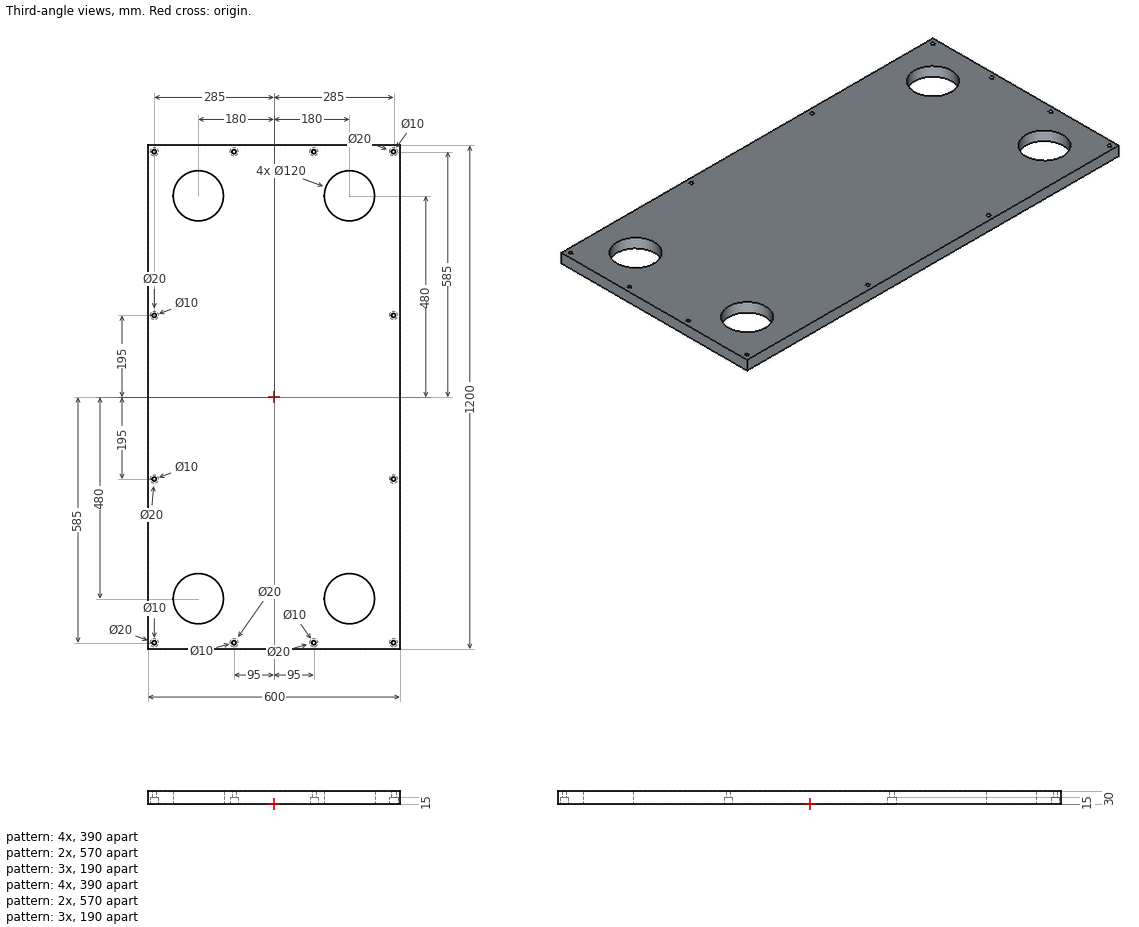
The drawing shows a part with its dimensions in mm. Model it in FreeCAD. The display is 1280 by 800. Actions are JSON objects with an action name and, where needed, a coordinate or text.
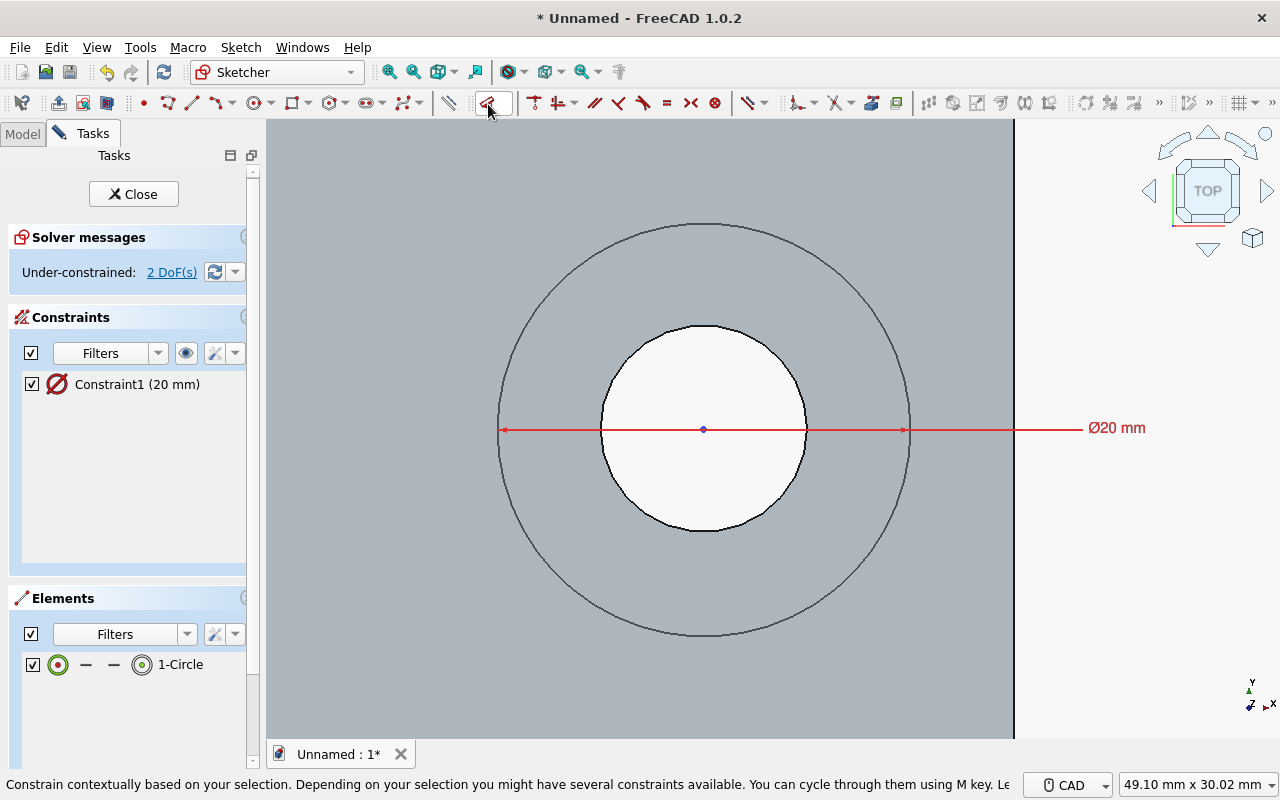
{"action": "left_click", "coordinate": [704, 430]}
{"action": "left_click", "coordinate": [405, 396]}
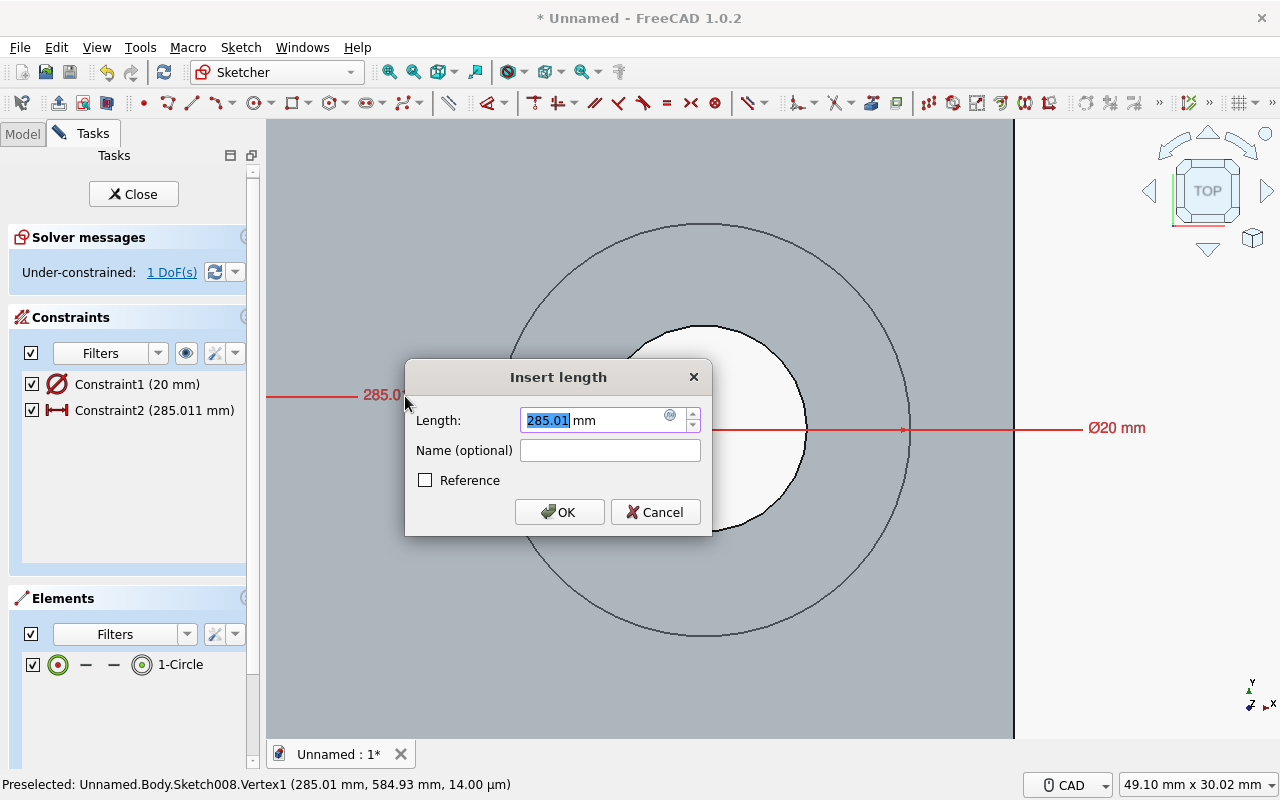
{"action": "type", "text": "285"}
{"action": "key", "text": "Return"}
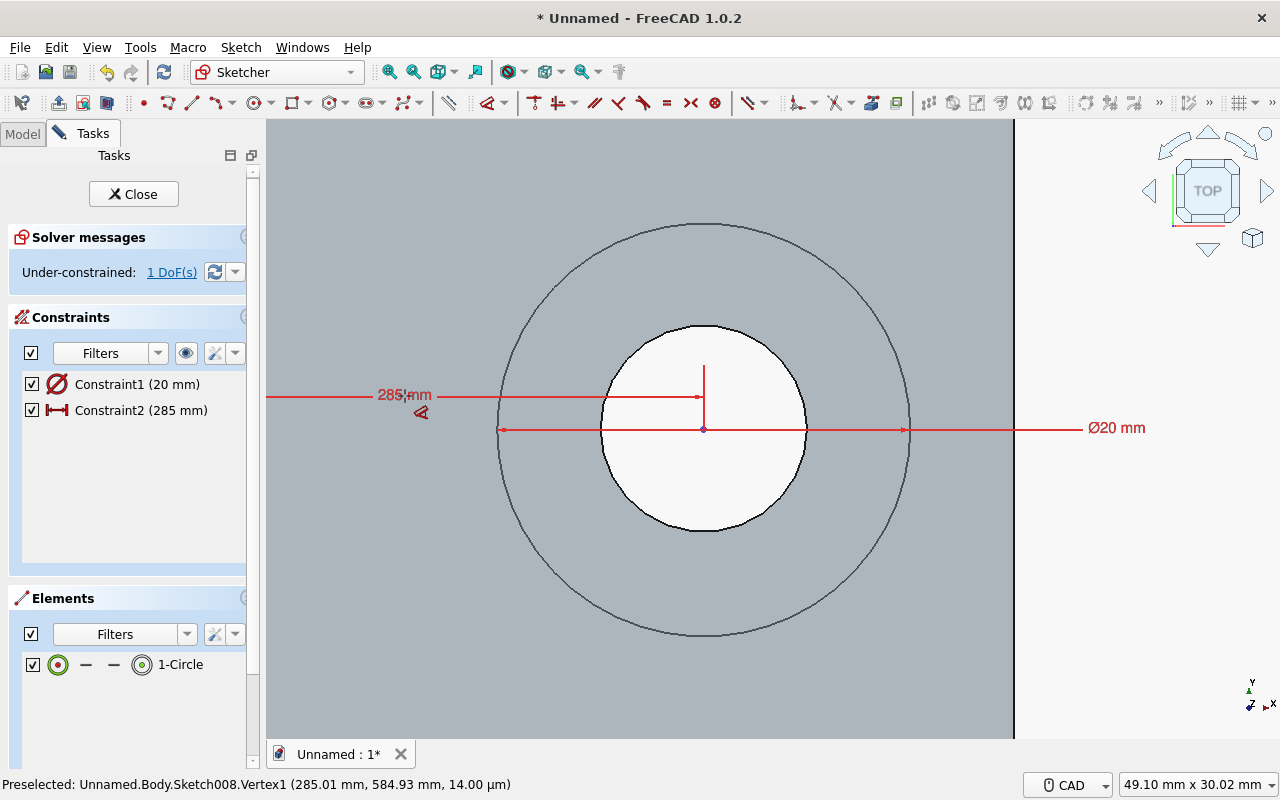
{"action": "left_click", "coordinate": [704, 430]}
{"action": "left_click", "coordinate": [738, 570]}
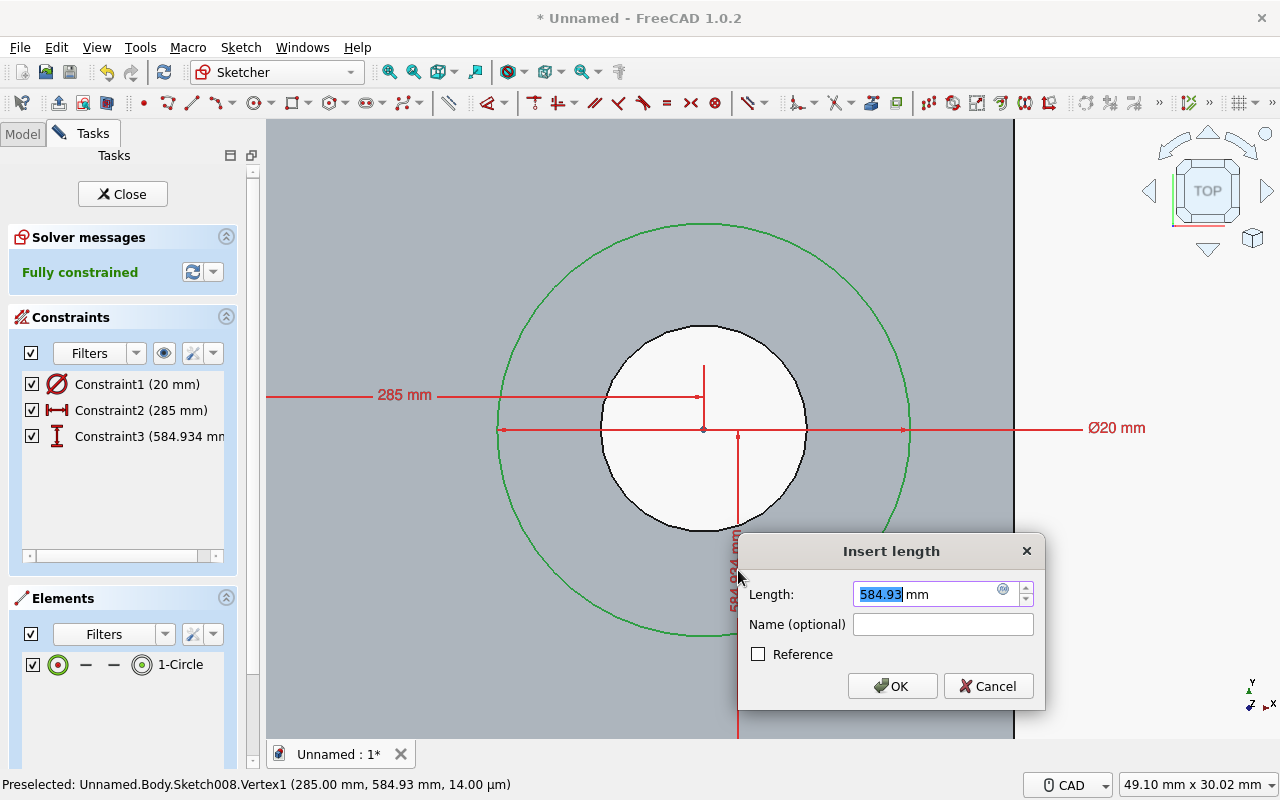
{"action": "type", "text": "585"}
{"action": "key", "text": "Return"}
{"action": "key", "text": "Escape"}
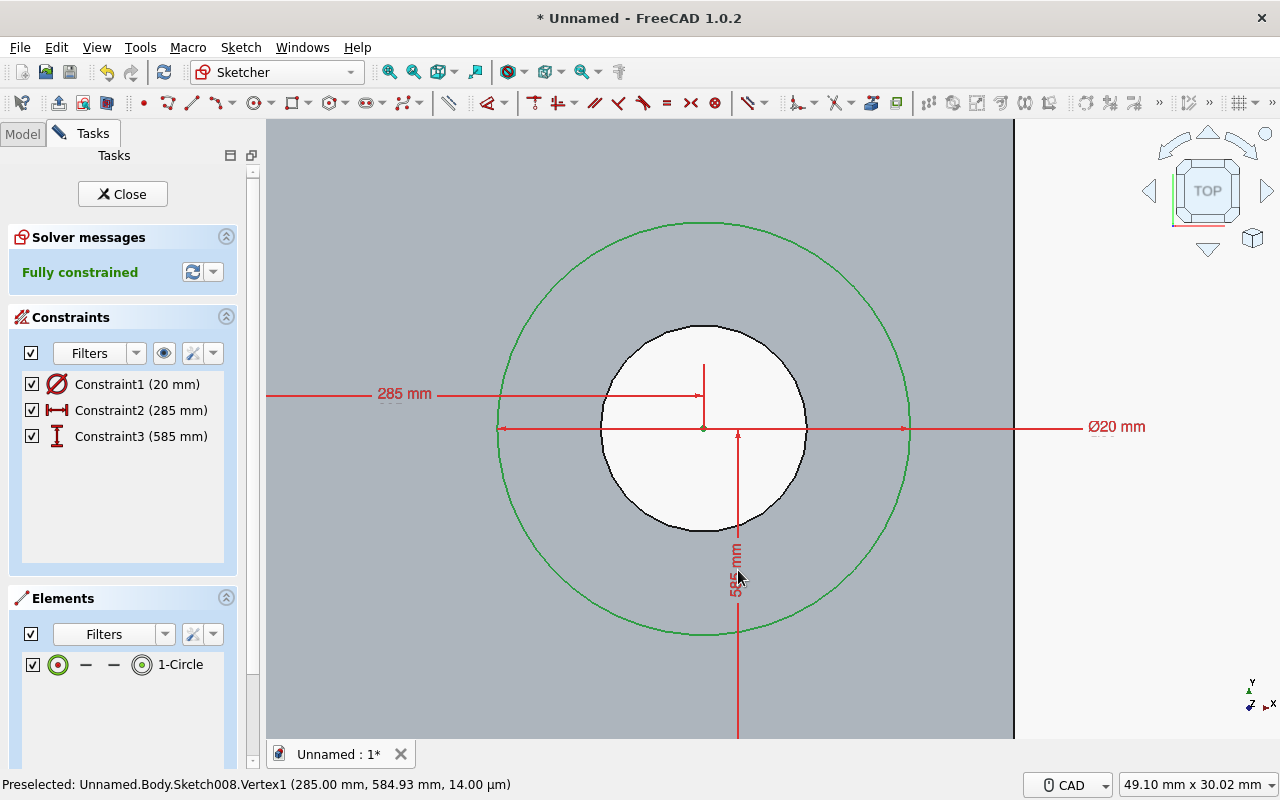
{"action": "left_click", "coordinate": [123, 194]}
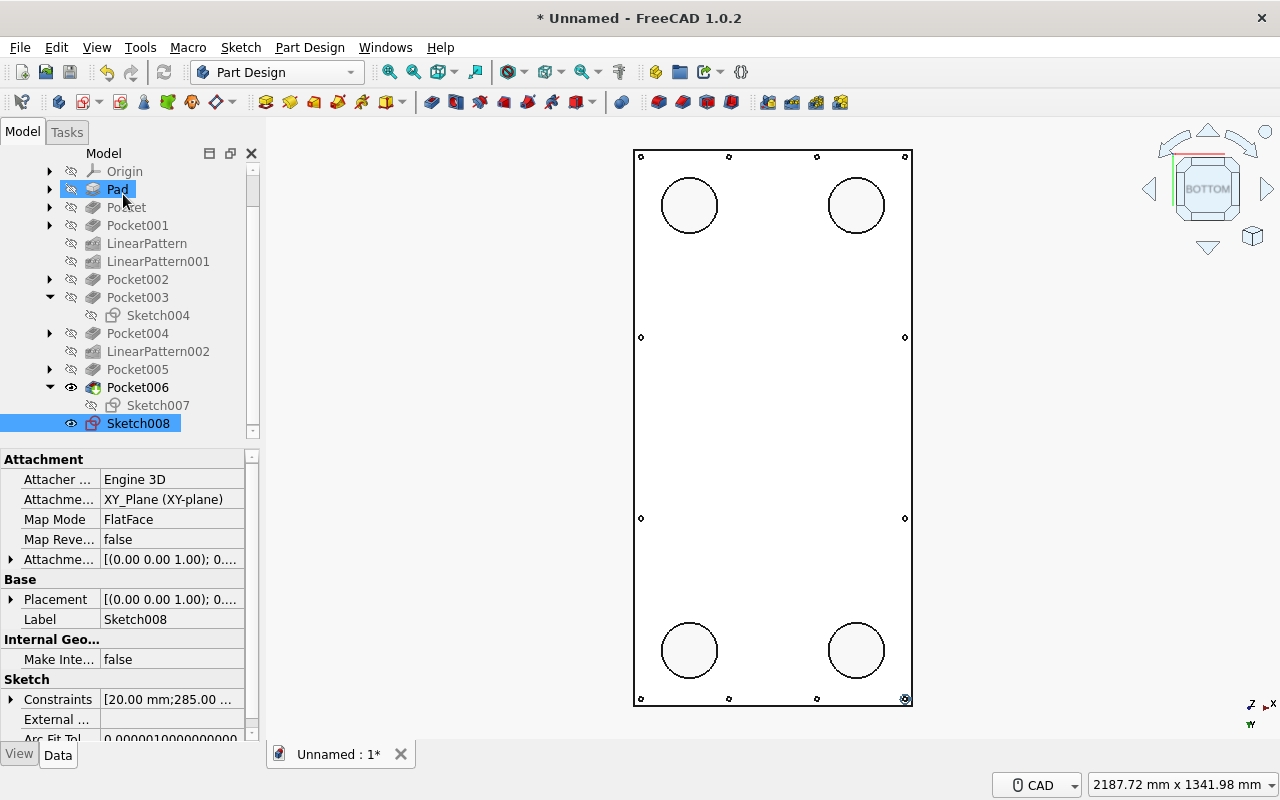
{"action": "left_click", "coordinate": [432, 102]}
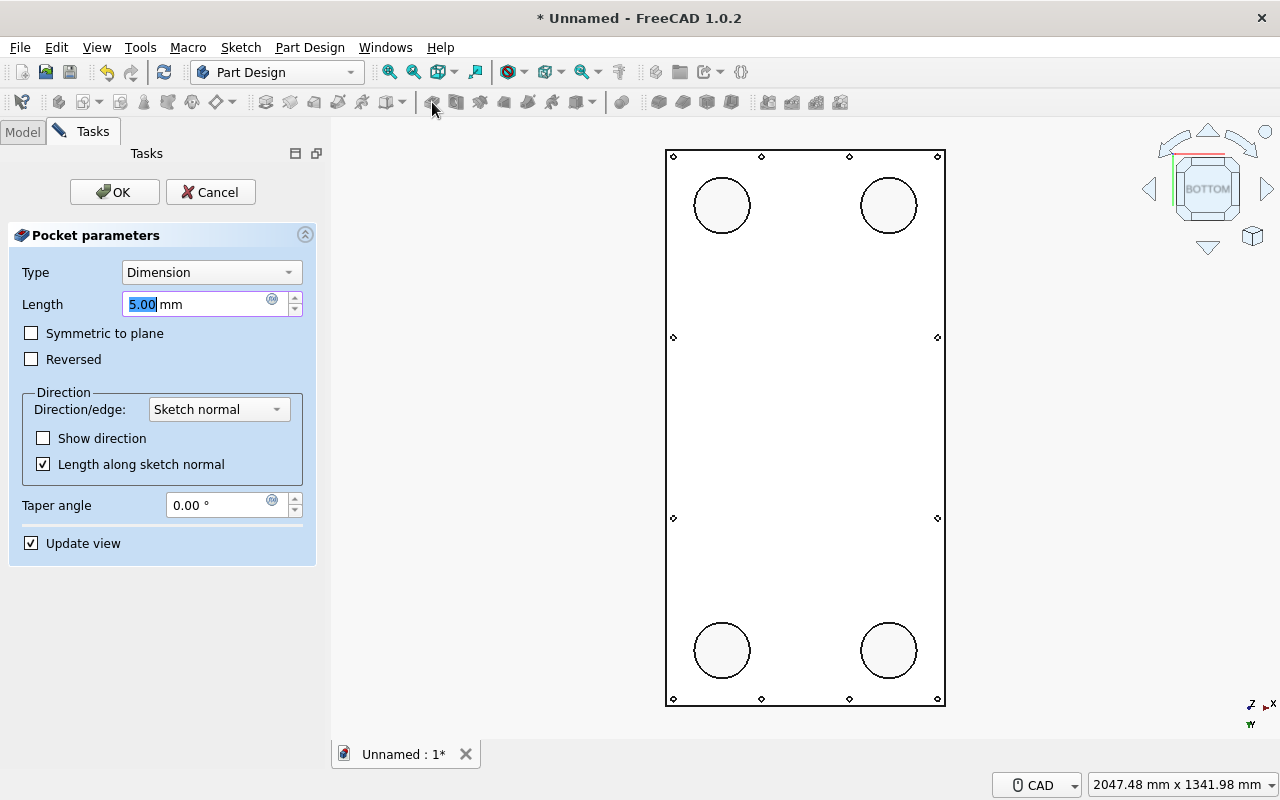
{"action": "type", "text": "15"}
{"action": "key", "text": "Tab"}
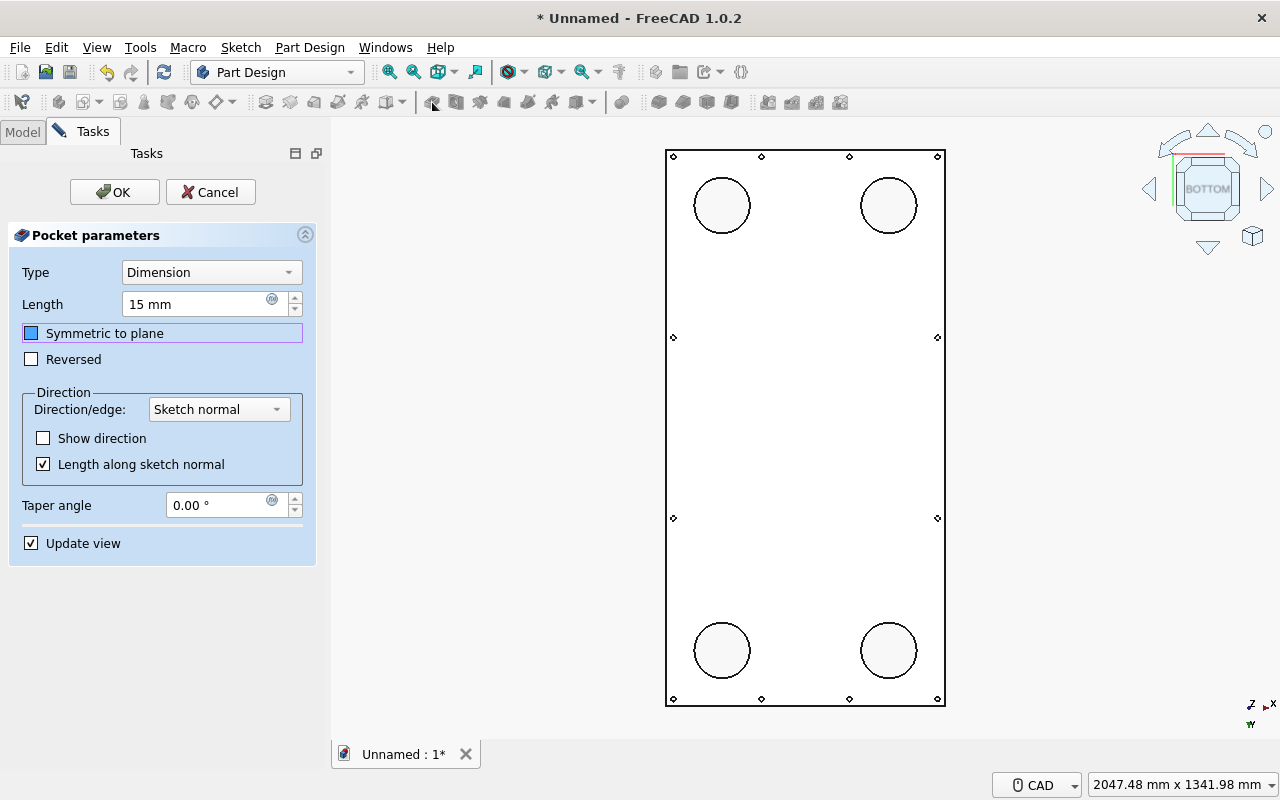
{"action": "left_click", "coordinate": [30, 359]}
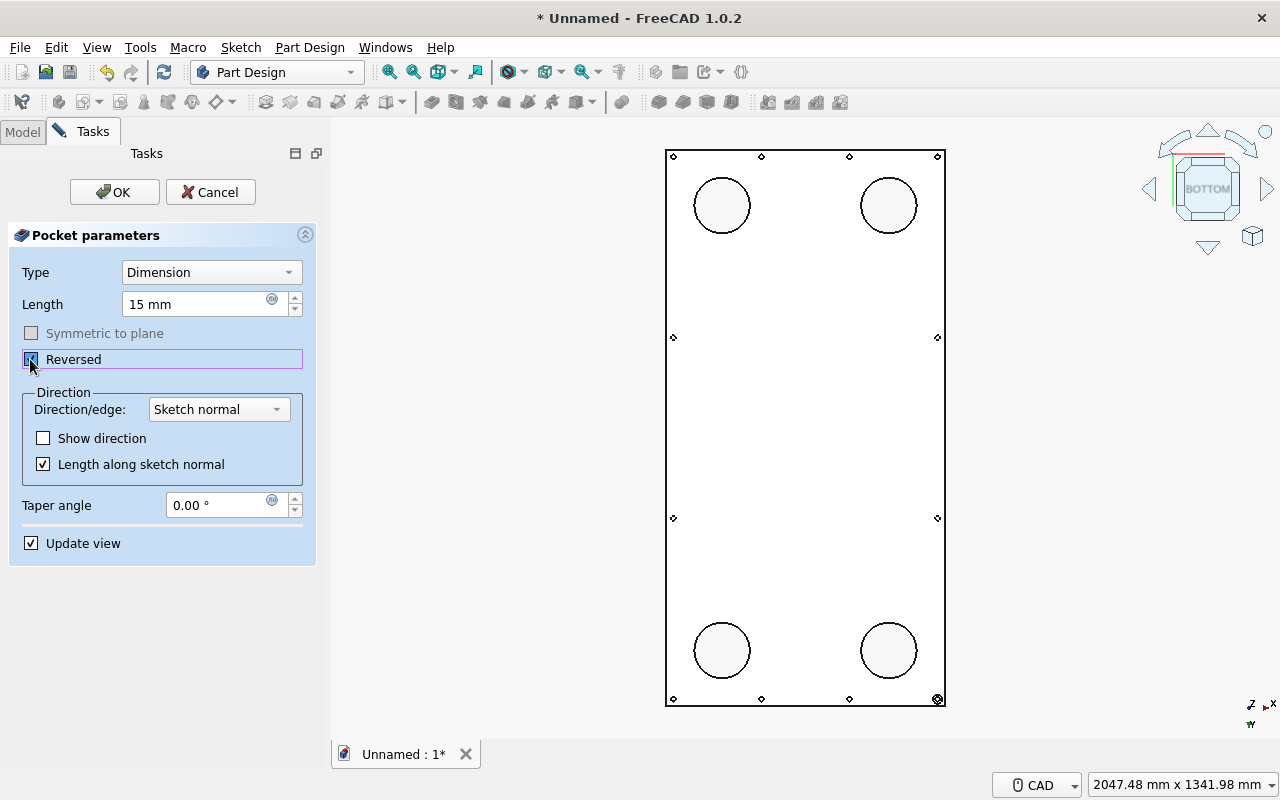
{"action": "left_click", "coordinate": [115, 192]}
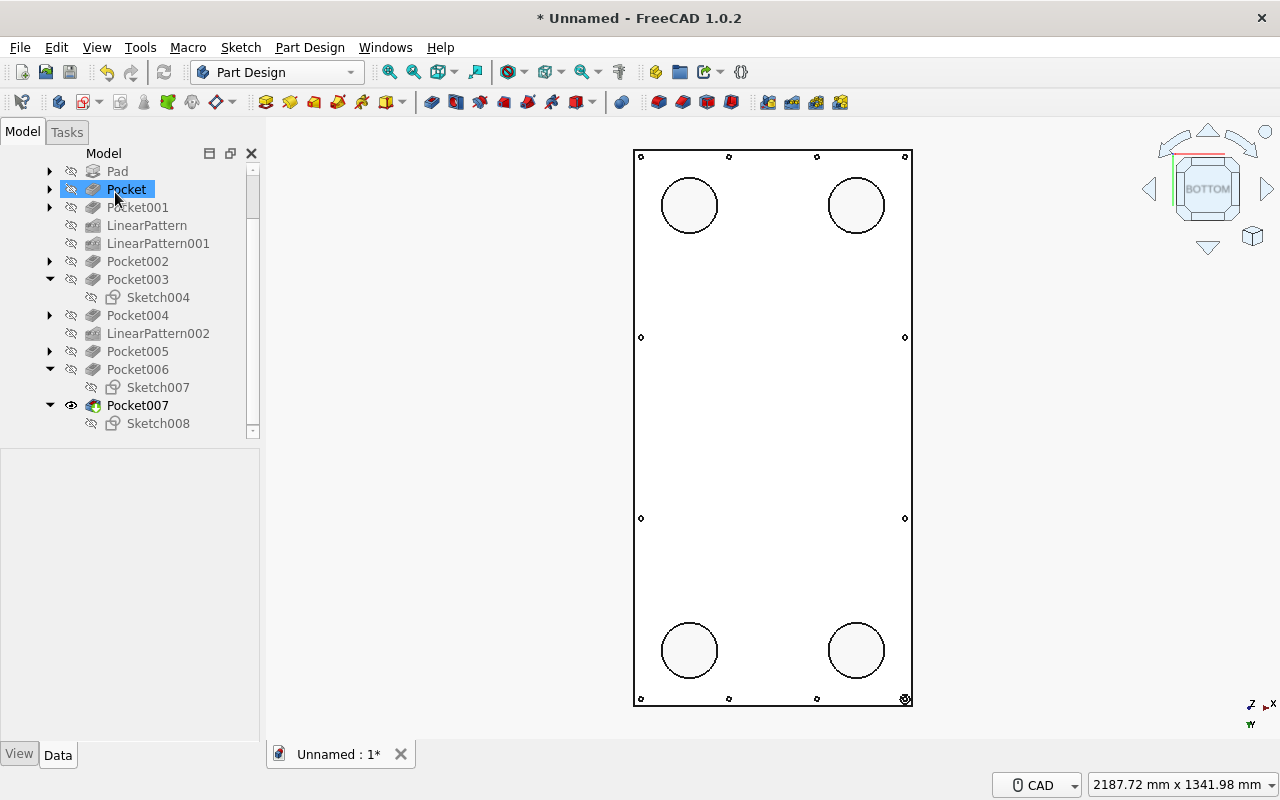
{"action": "left_click", "coordinate": [116, 405]}